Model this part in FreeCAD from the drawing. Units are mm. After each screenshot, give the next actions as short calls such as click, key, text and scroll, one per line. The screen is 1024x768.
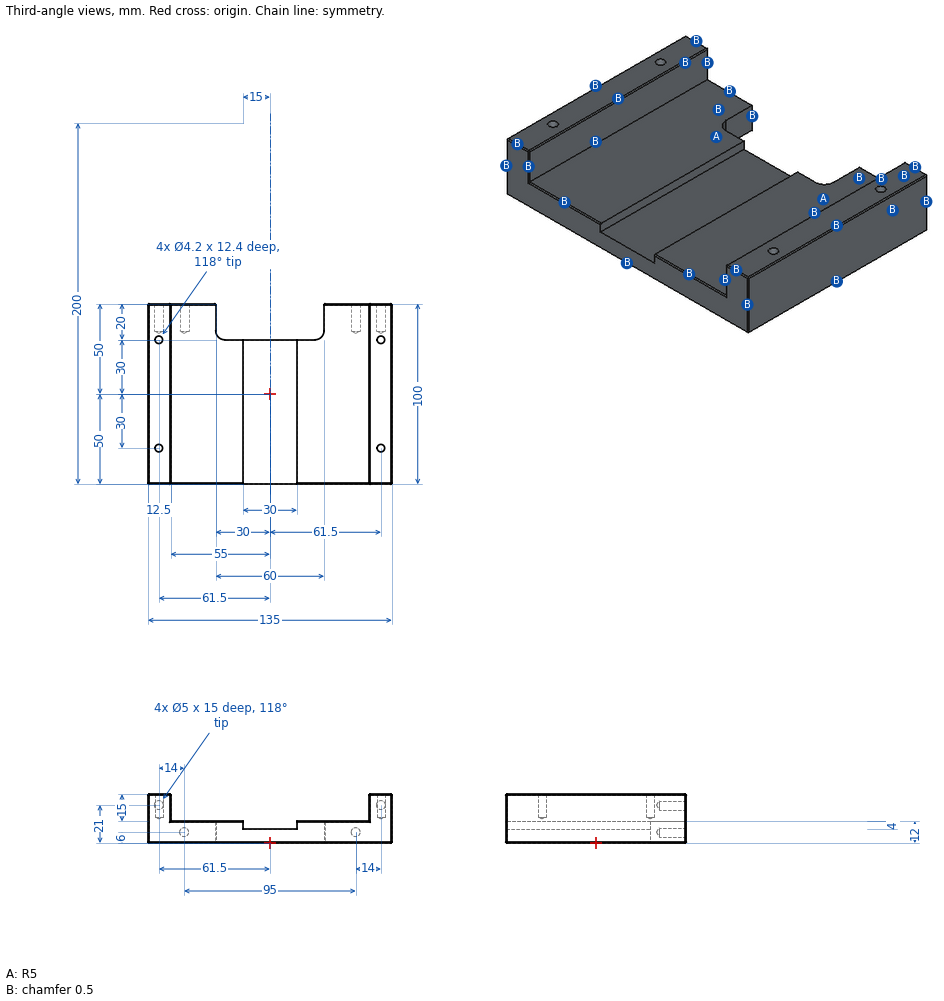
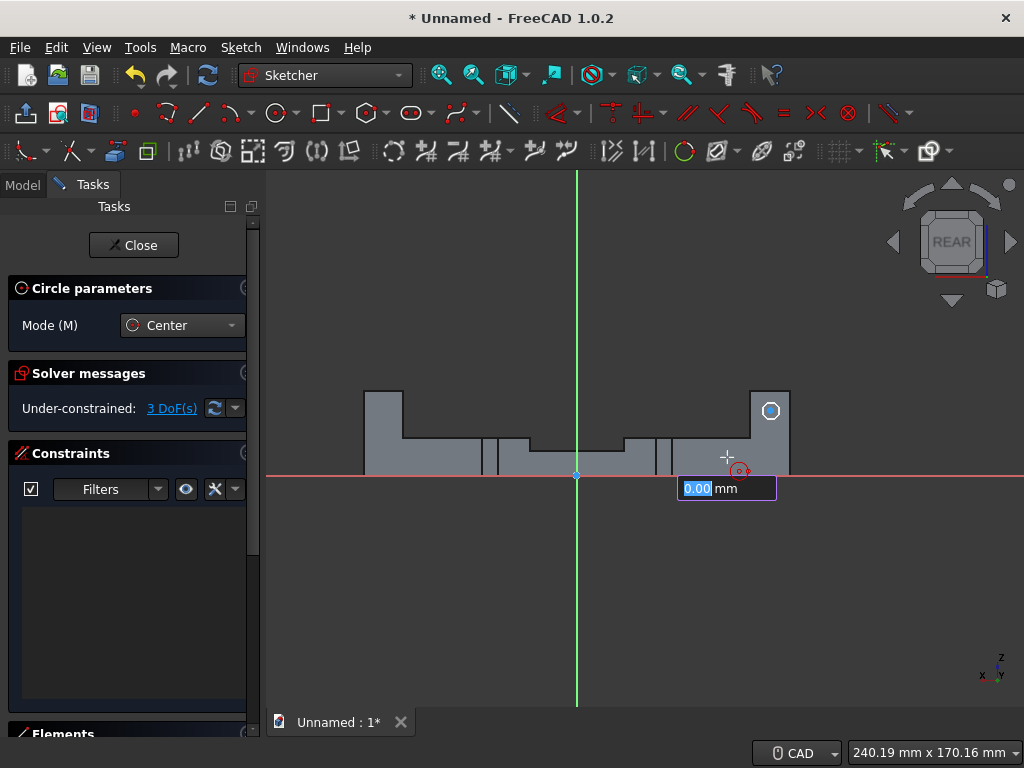
scroll(732, 451, up, 4)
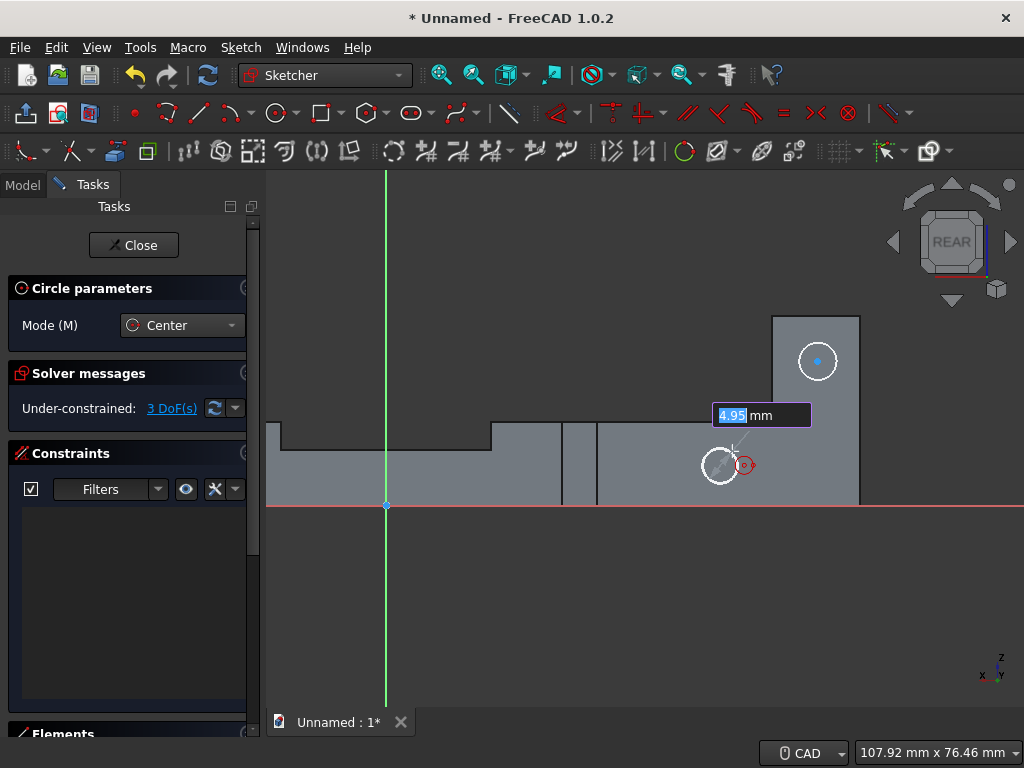
click(732, 451)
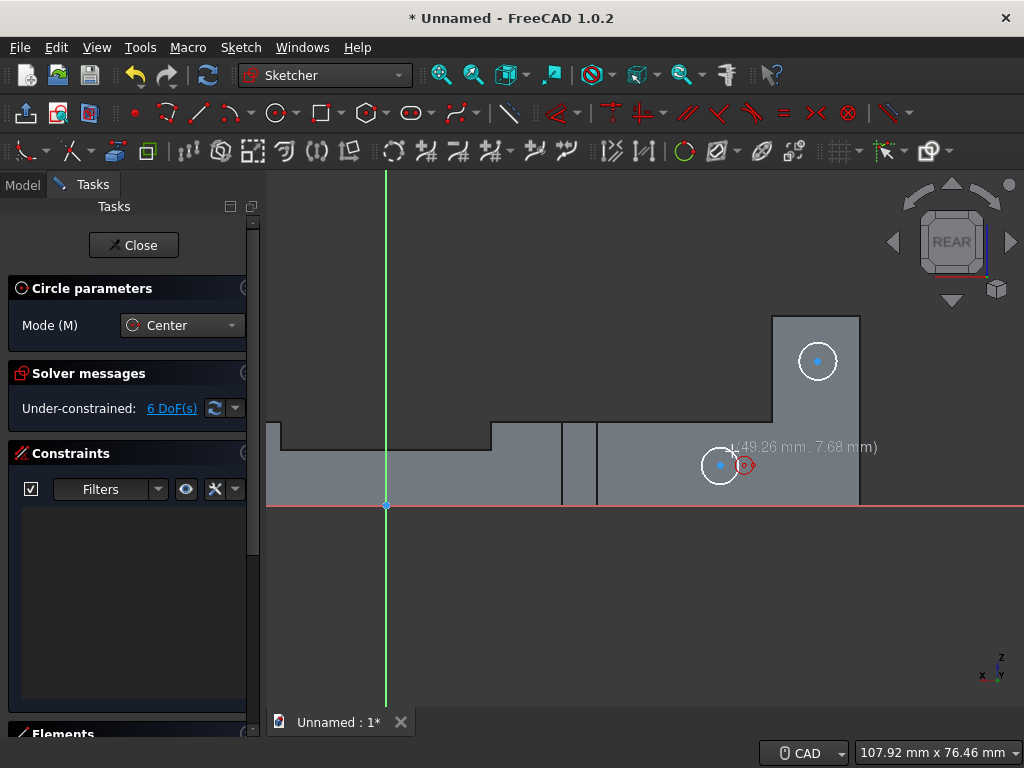
scroll(732, 451, down, 4)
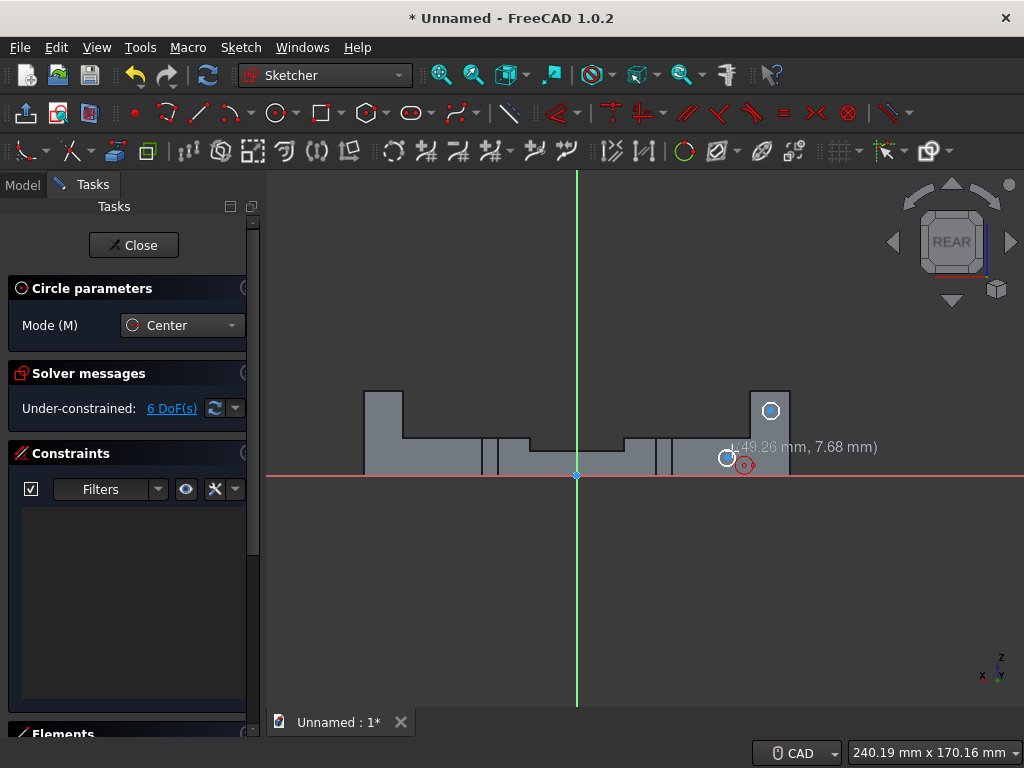
scroll(427, 457, up, 6)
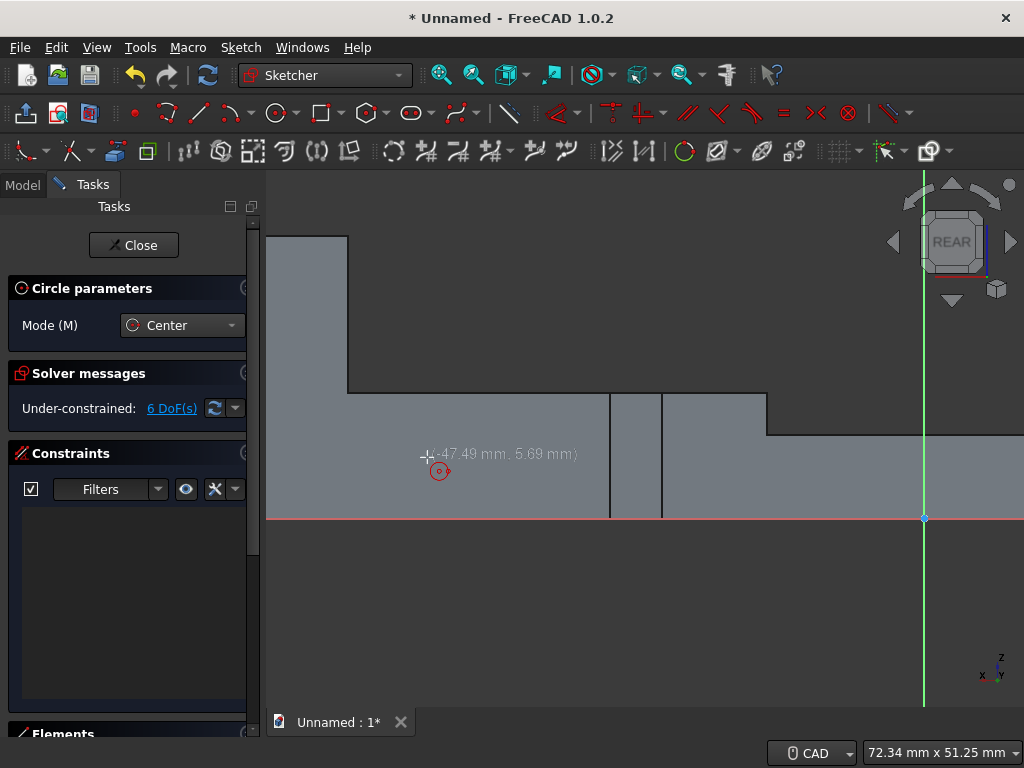
scroll(427, 457, down, 6)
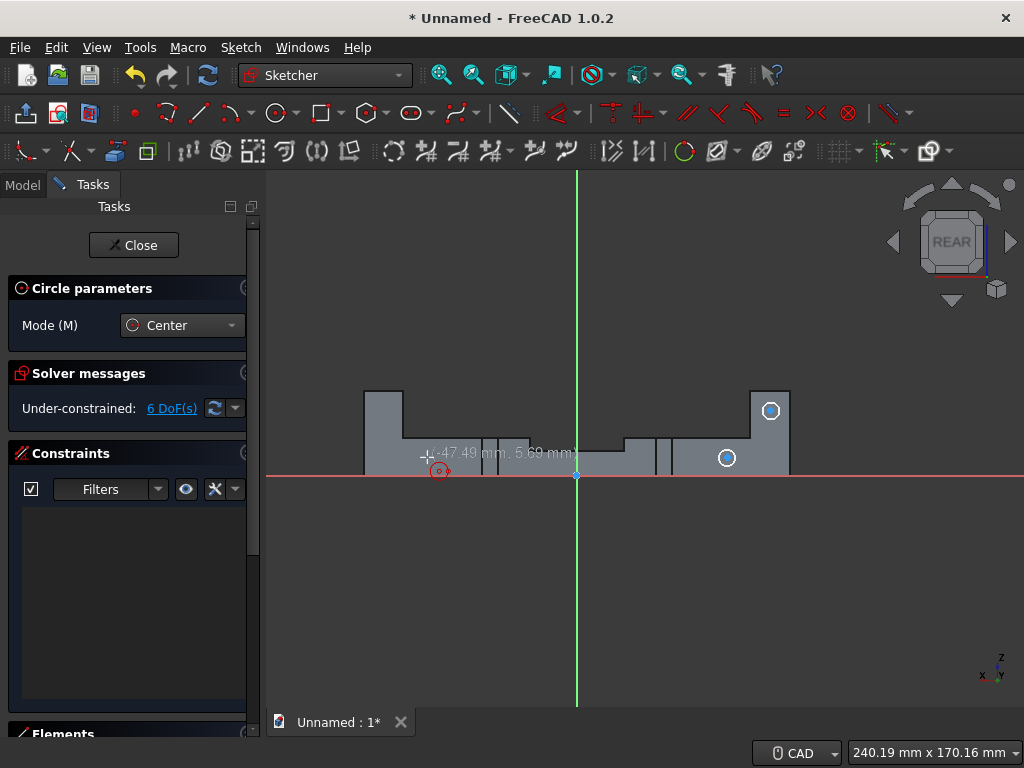
click(427, 457)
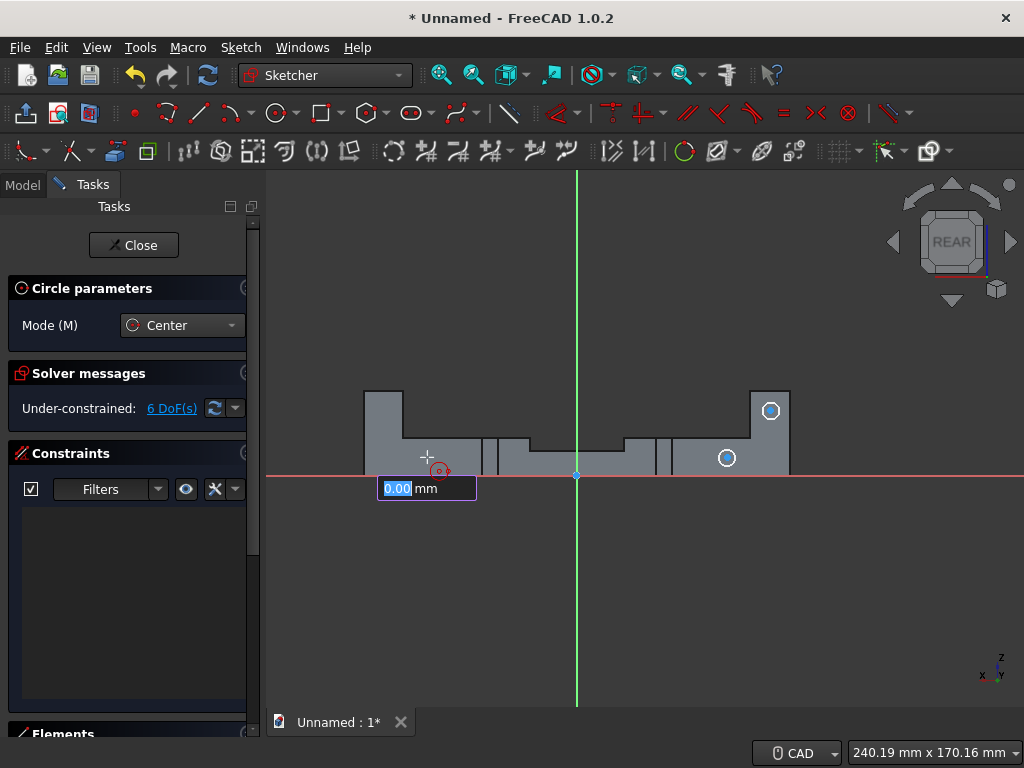
scroll(433, 451, up, 4)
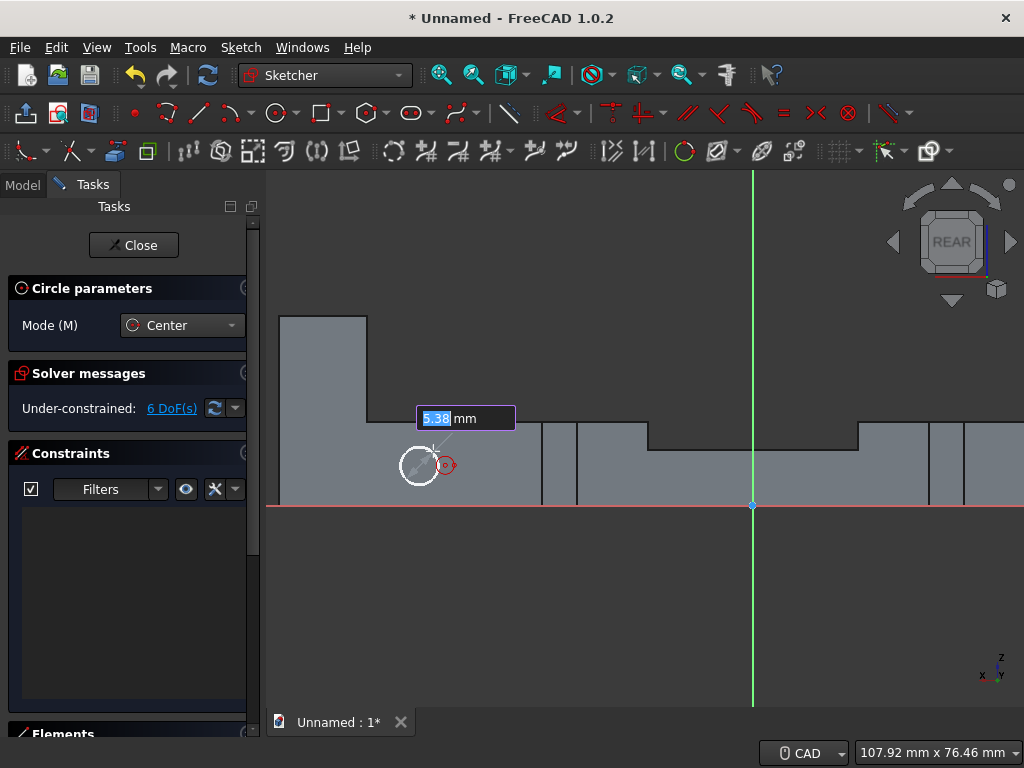
click(432, 451)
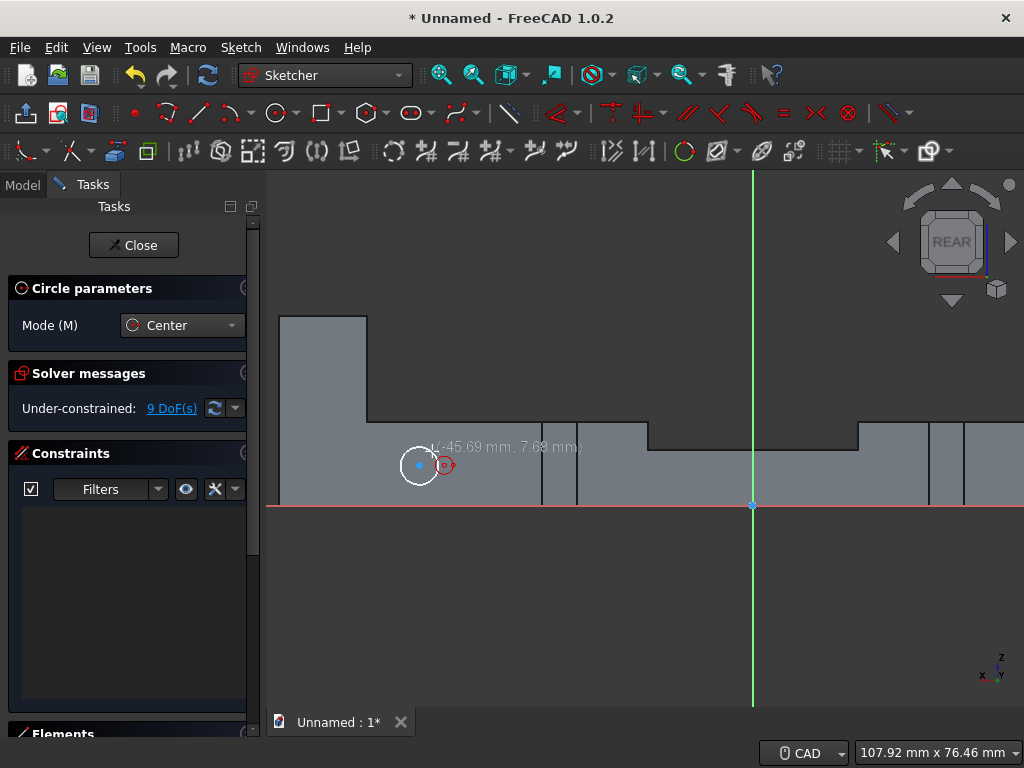
scroll(321, 358, up, 2)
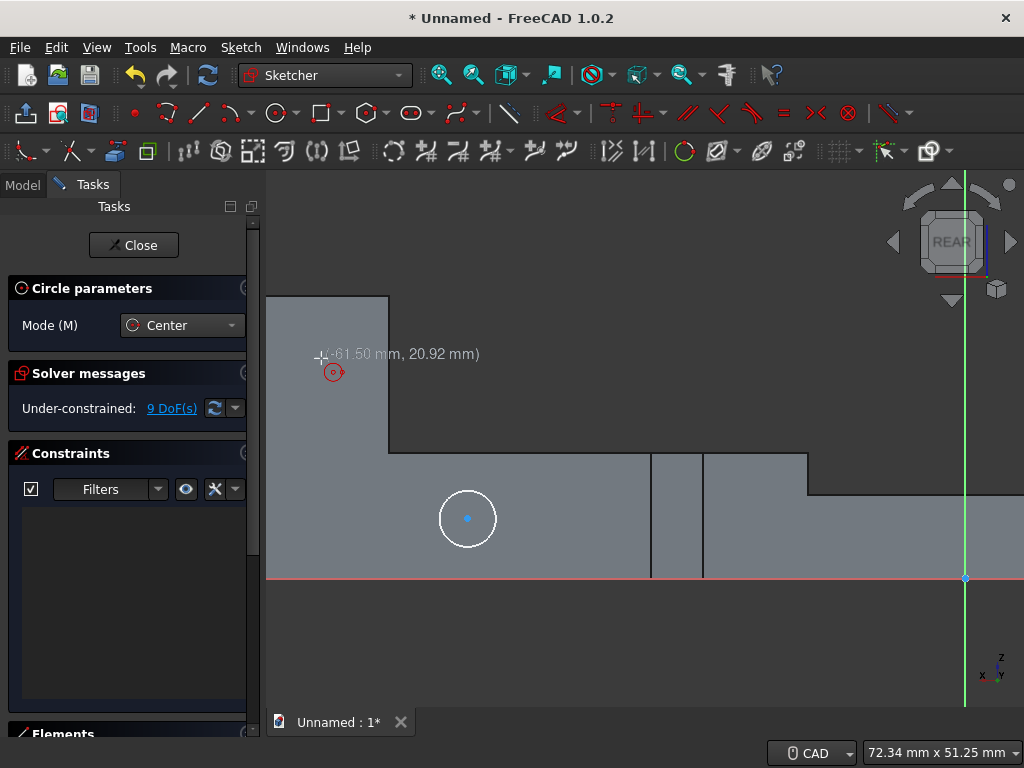
scroll(409, 431, down, 6)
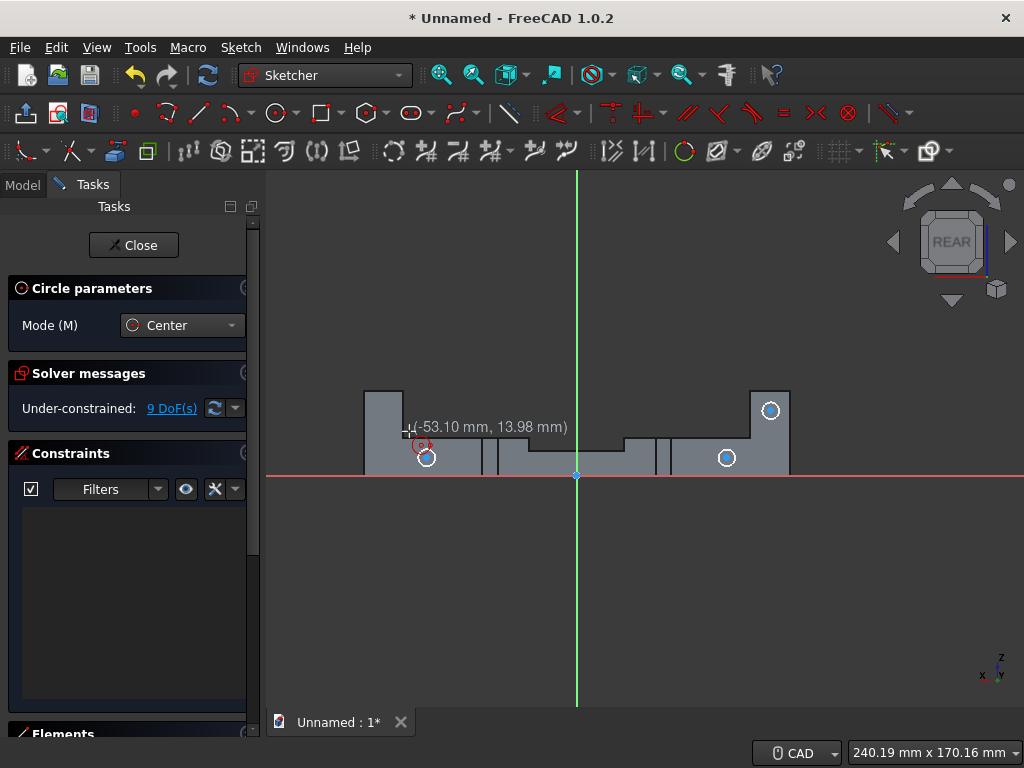
click(383, 409)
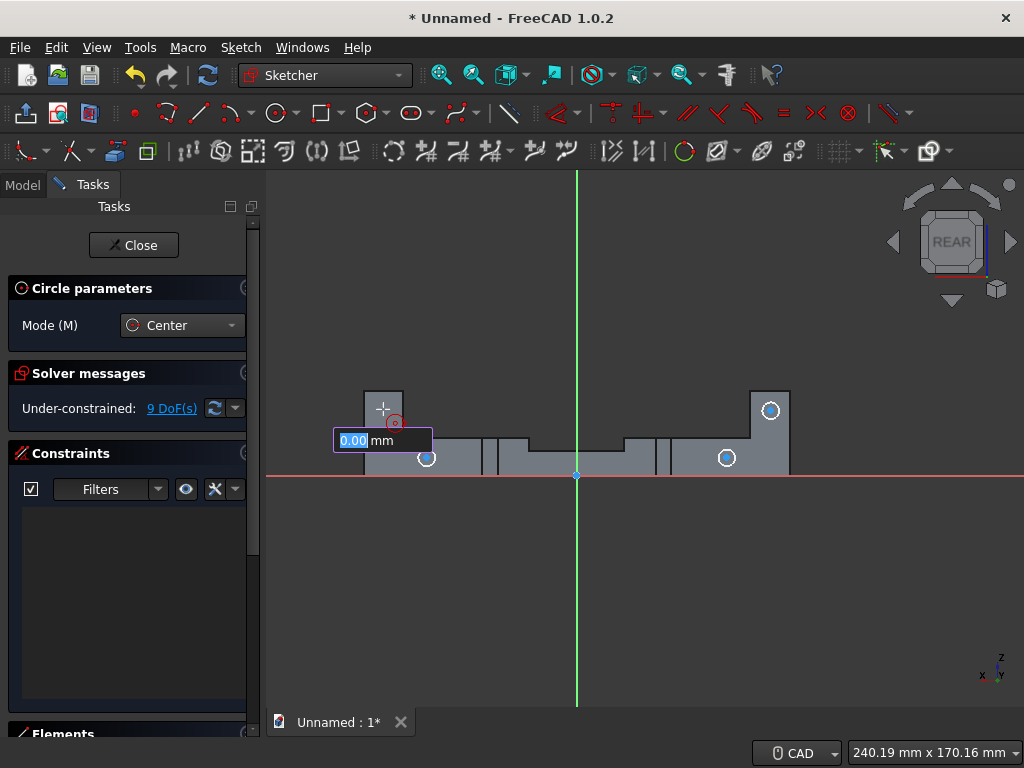
scroll(388, 404, up, 4)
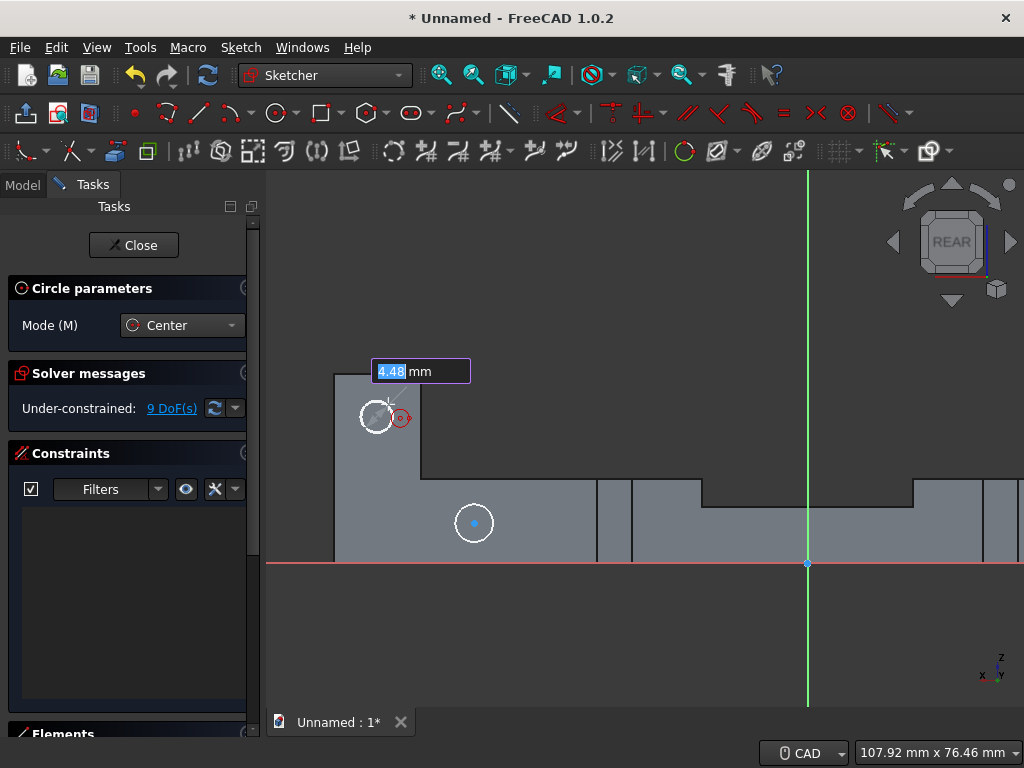
click(388, 403)
key(Escape)